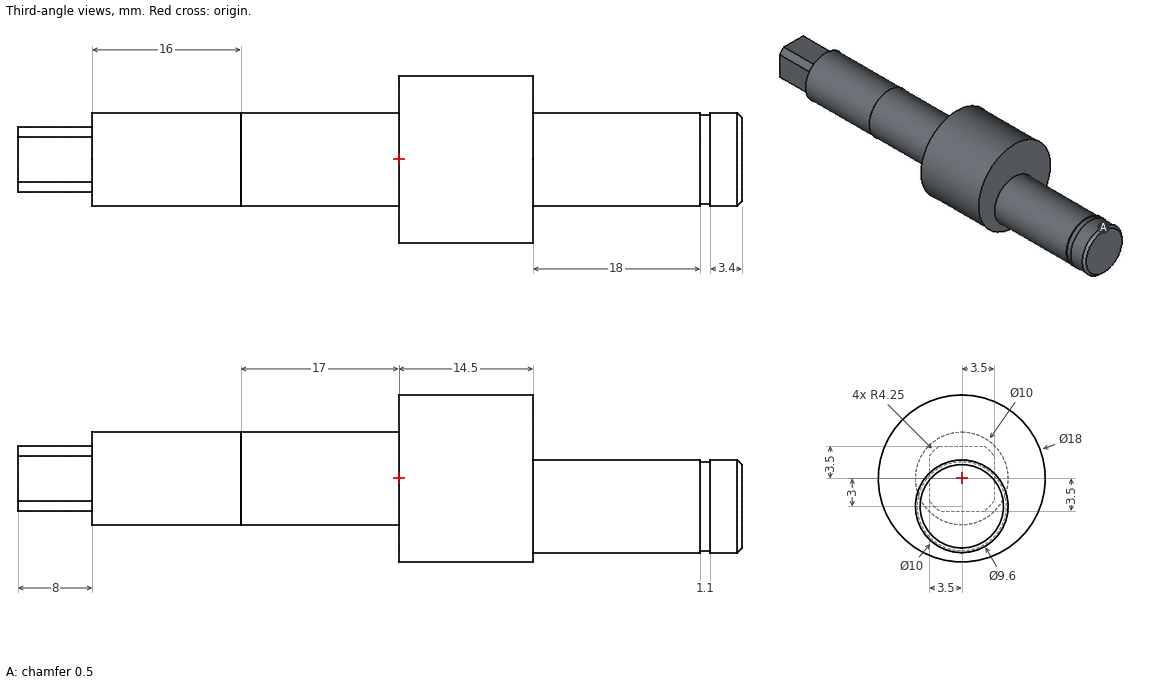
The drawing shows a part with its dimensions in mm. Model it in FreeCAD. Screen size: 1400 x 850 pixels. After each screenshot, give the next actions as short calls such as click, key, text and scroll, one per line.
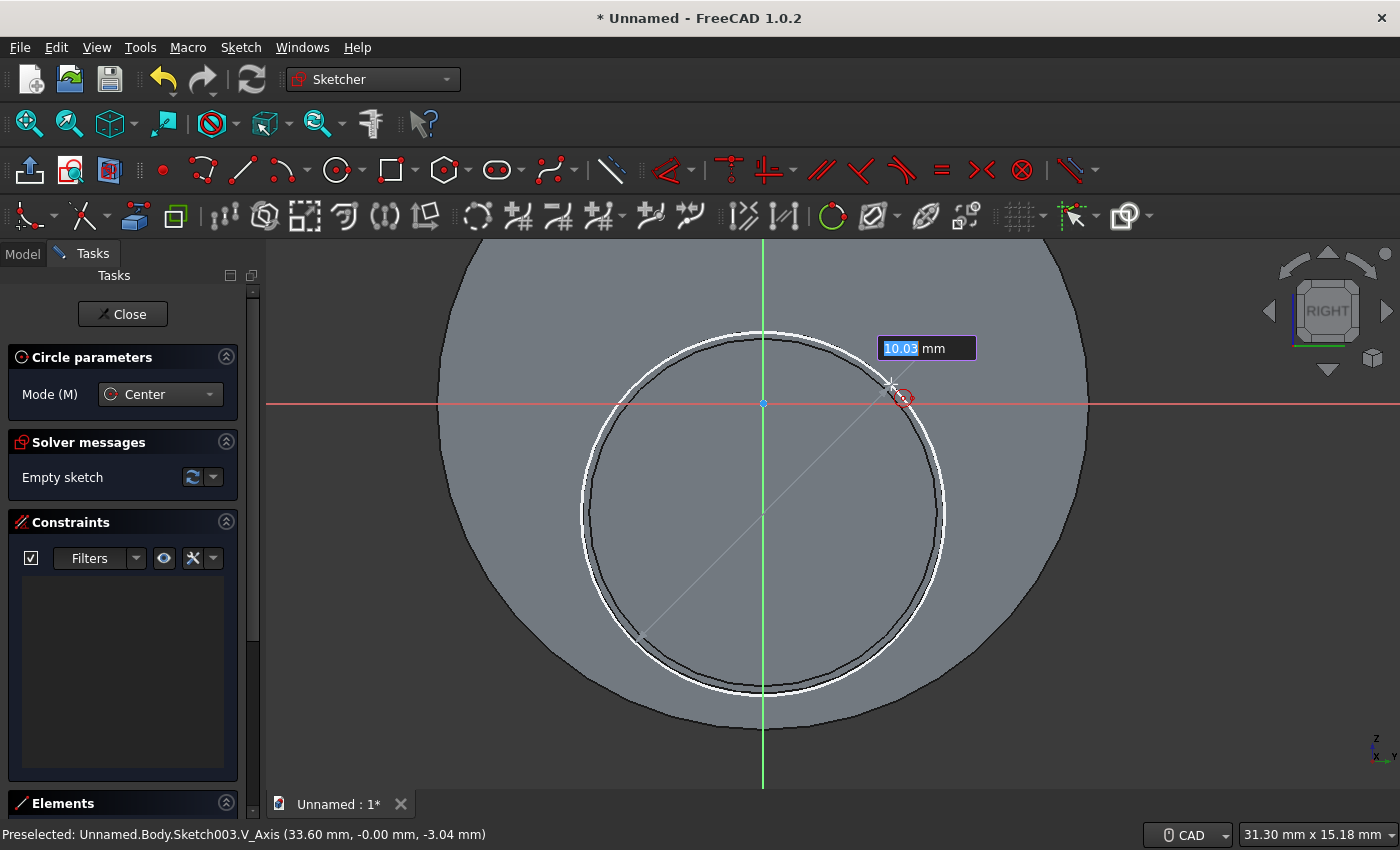
text(10)
key(Return)
key(Escape)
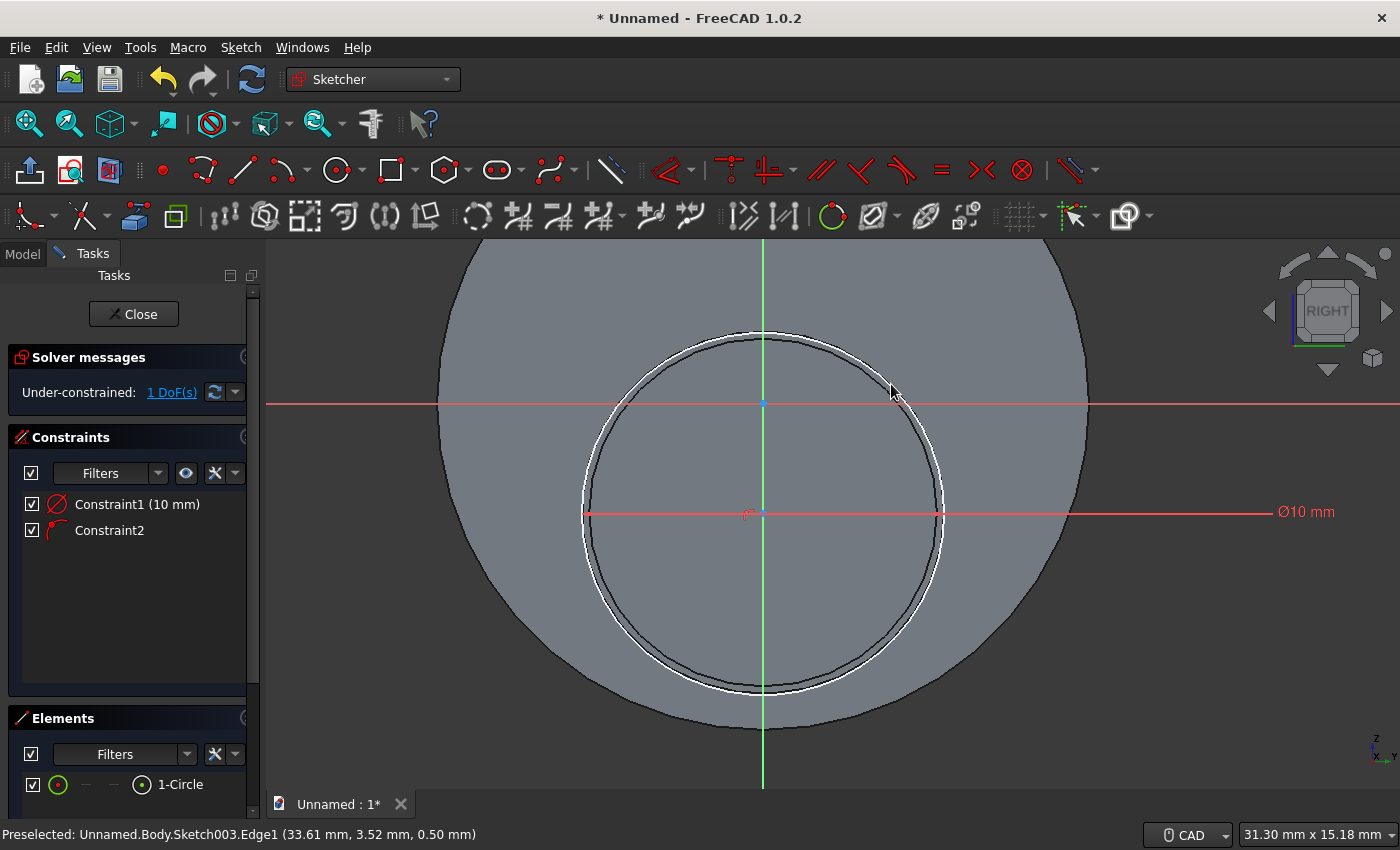
click(666, 170)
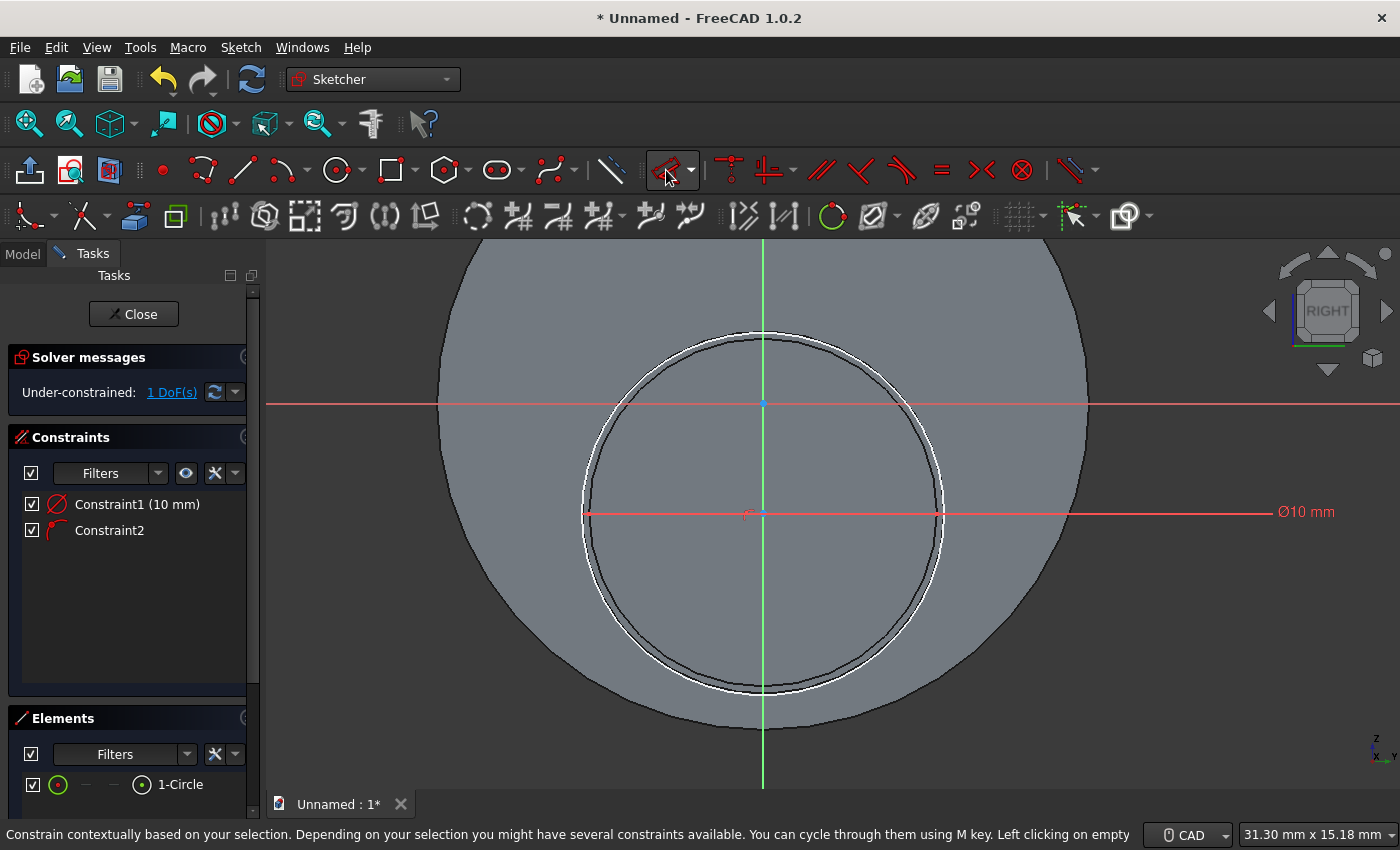
click(763, 514)
click(797, 459)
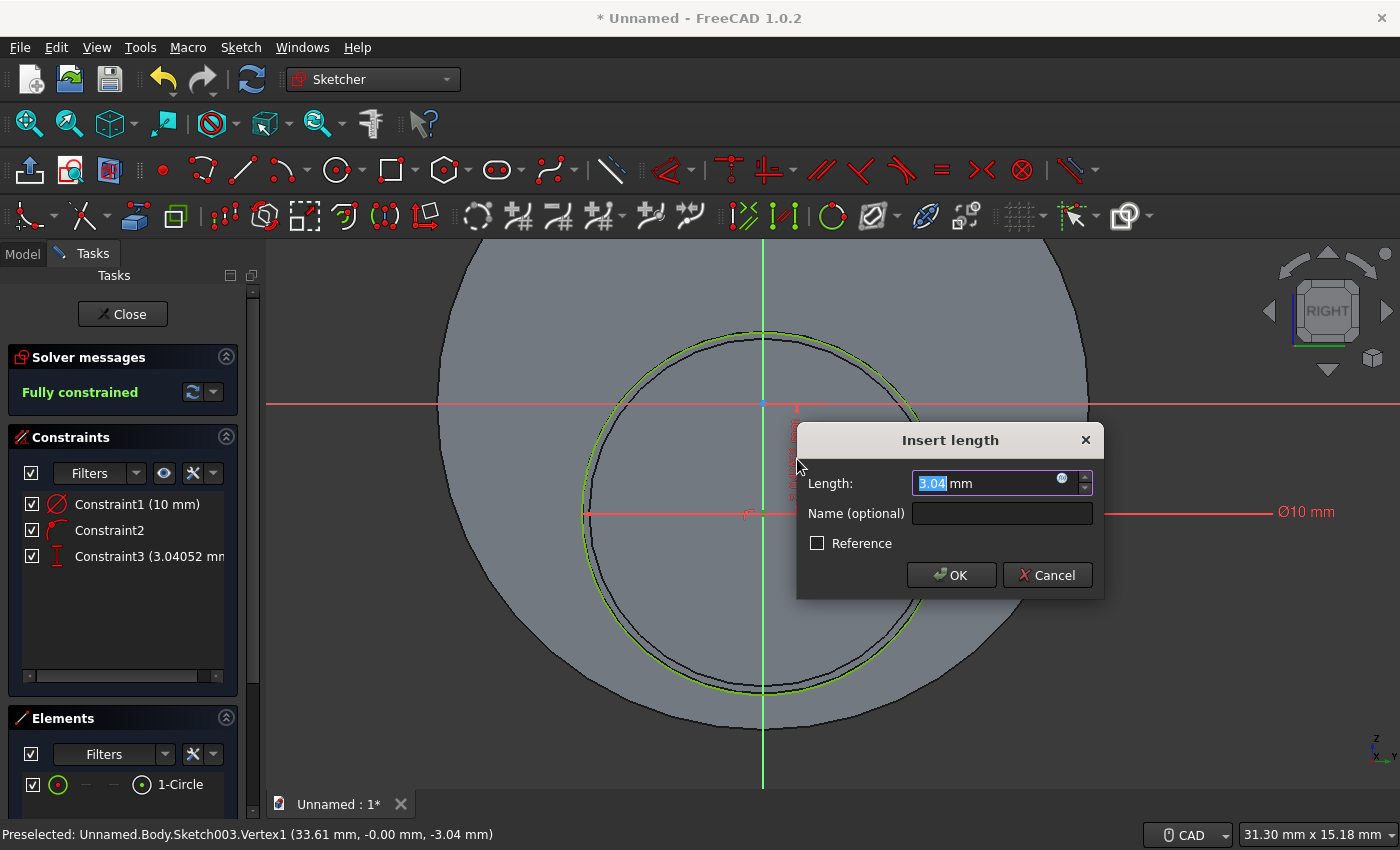
text(3)
key(Return)
key(Escape)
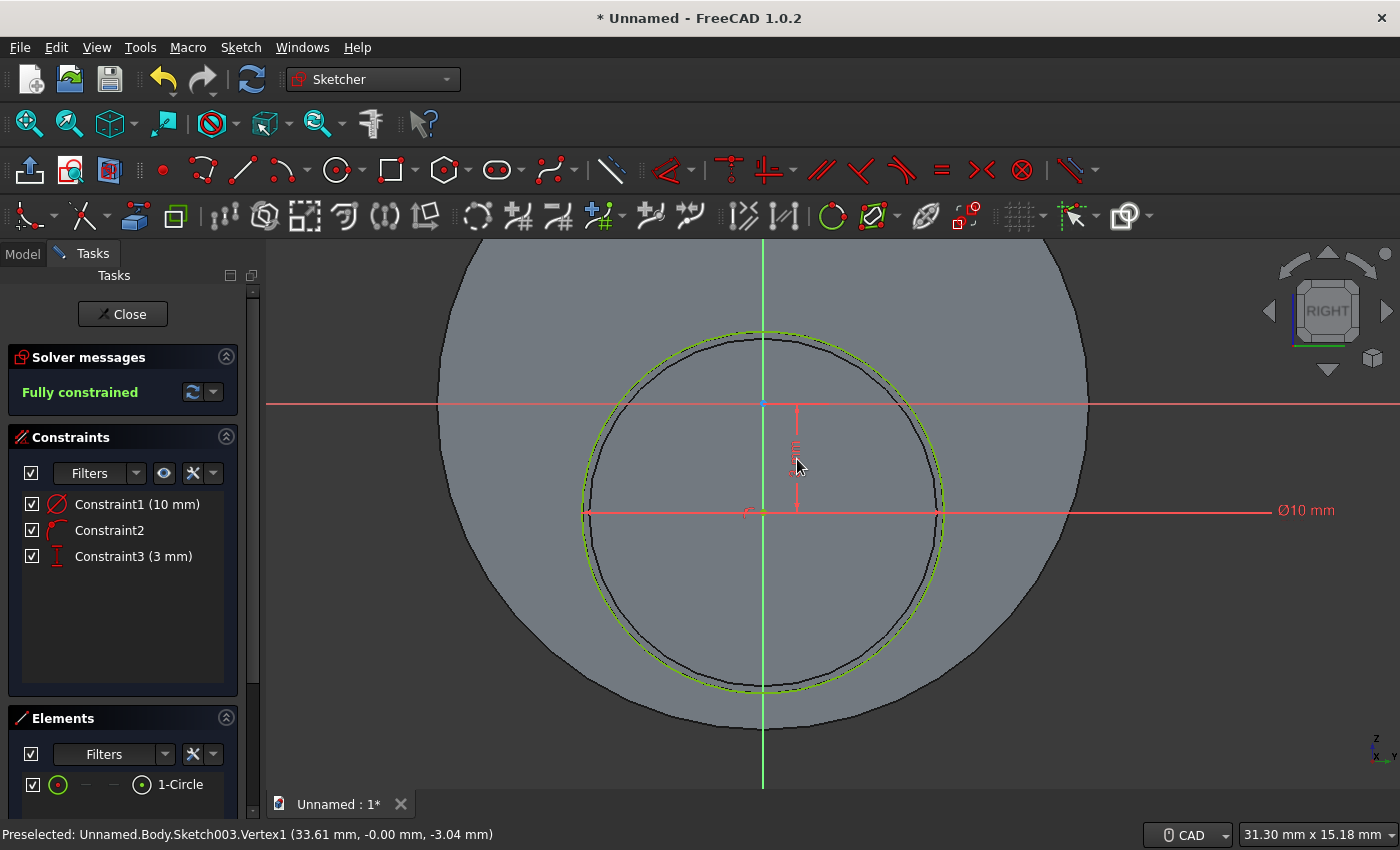
click(123, 314)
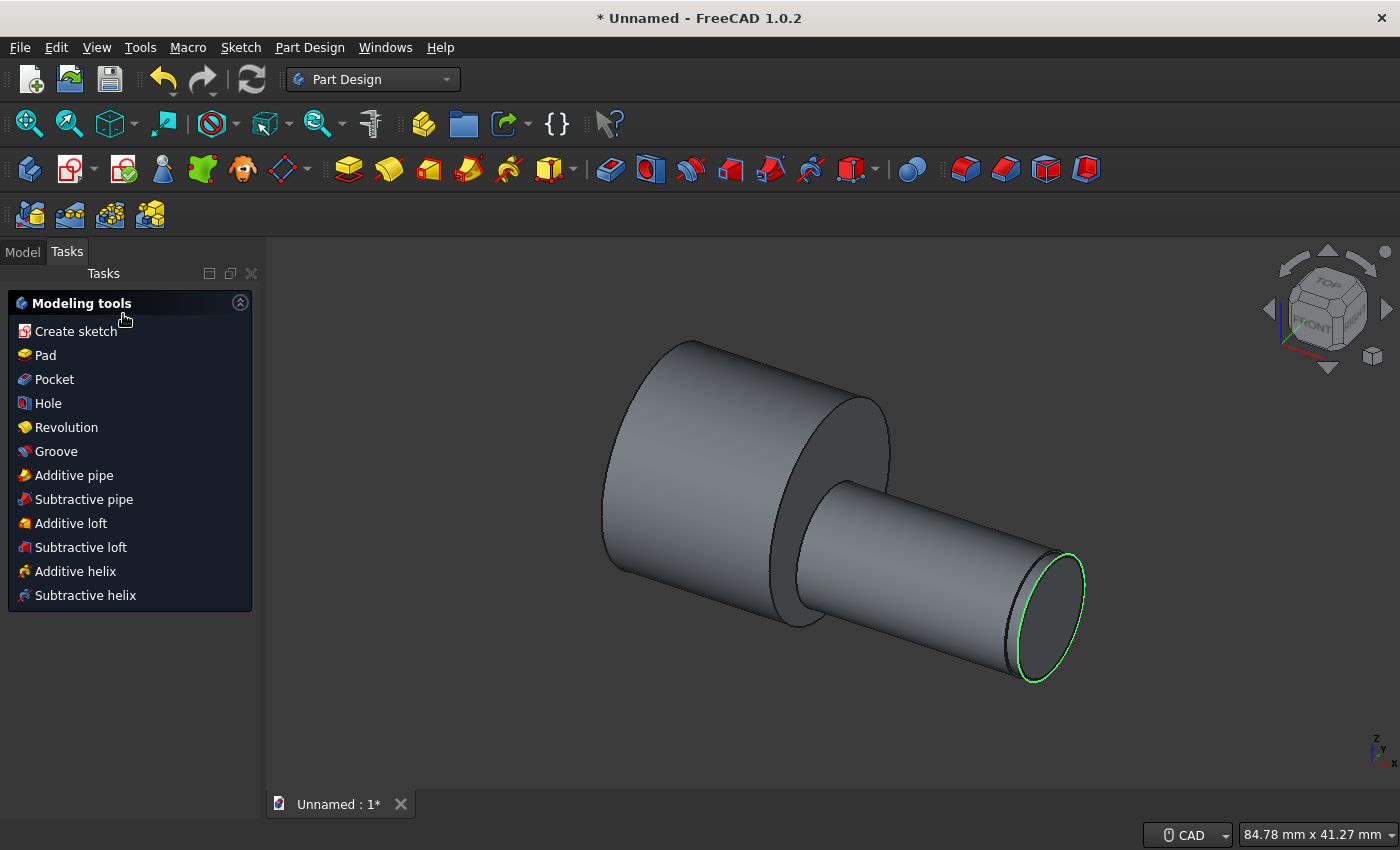
click(350, 170)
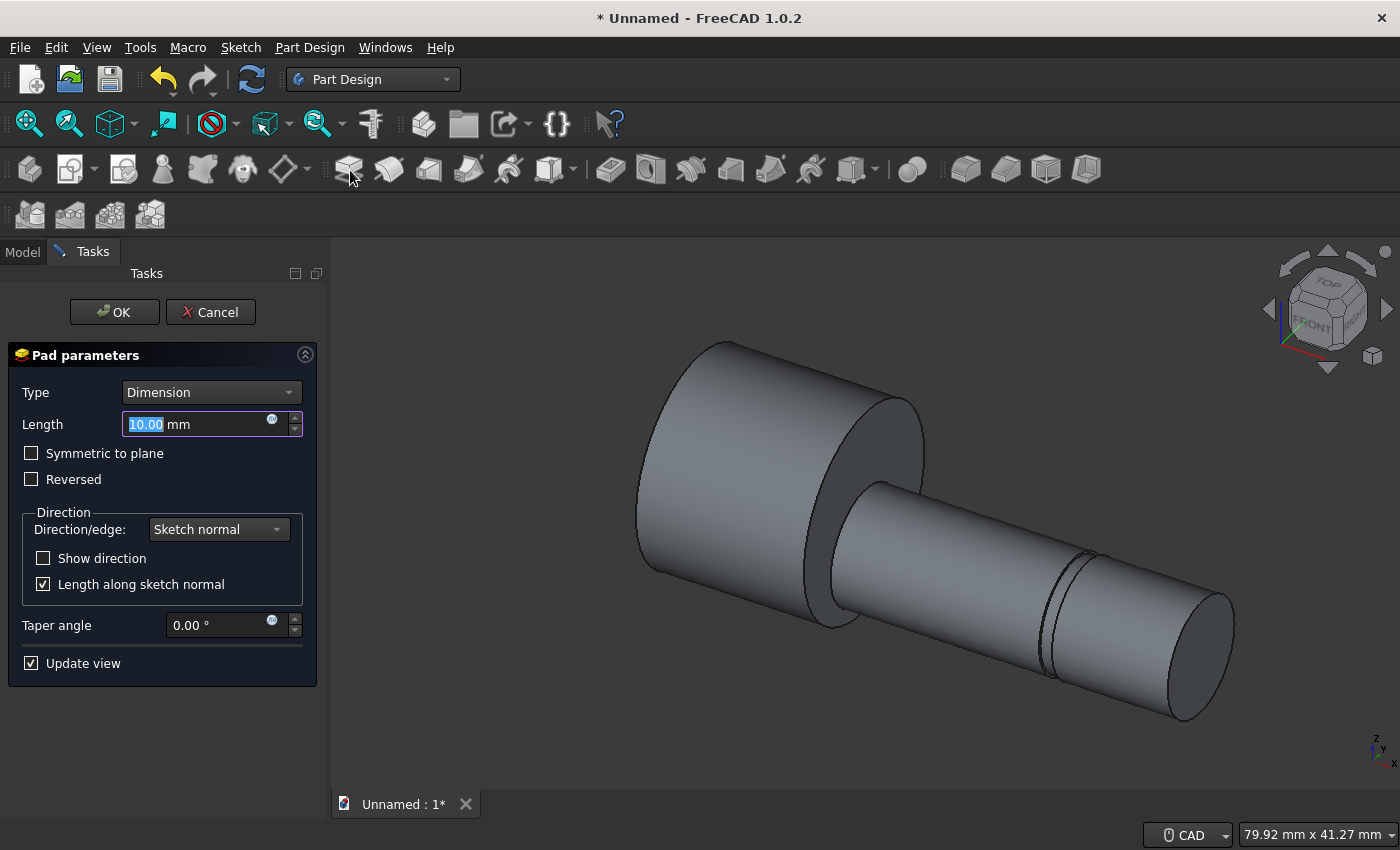
text(3.4)
key(Tab)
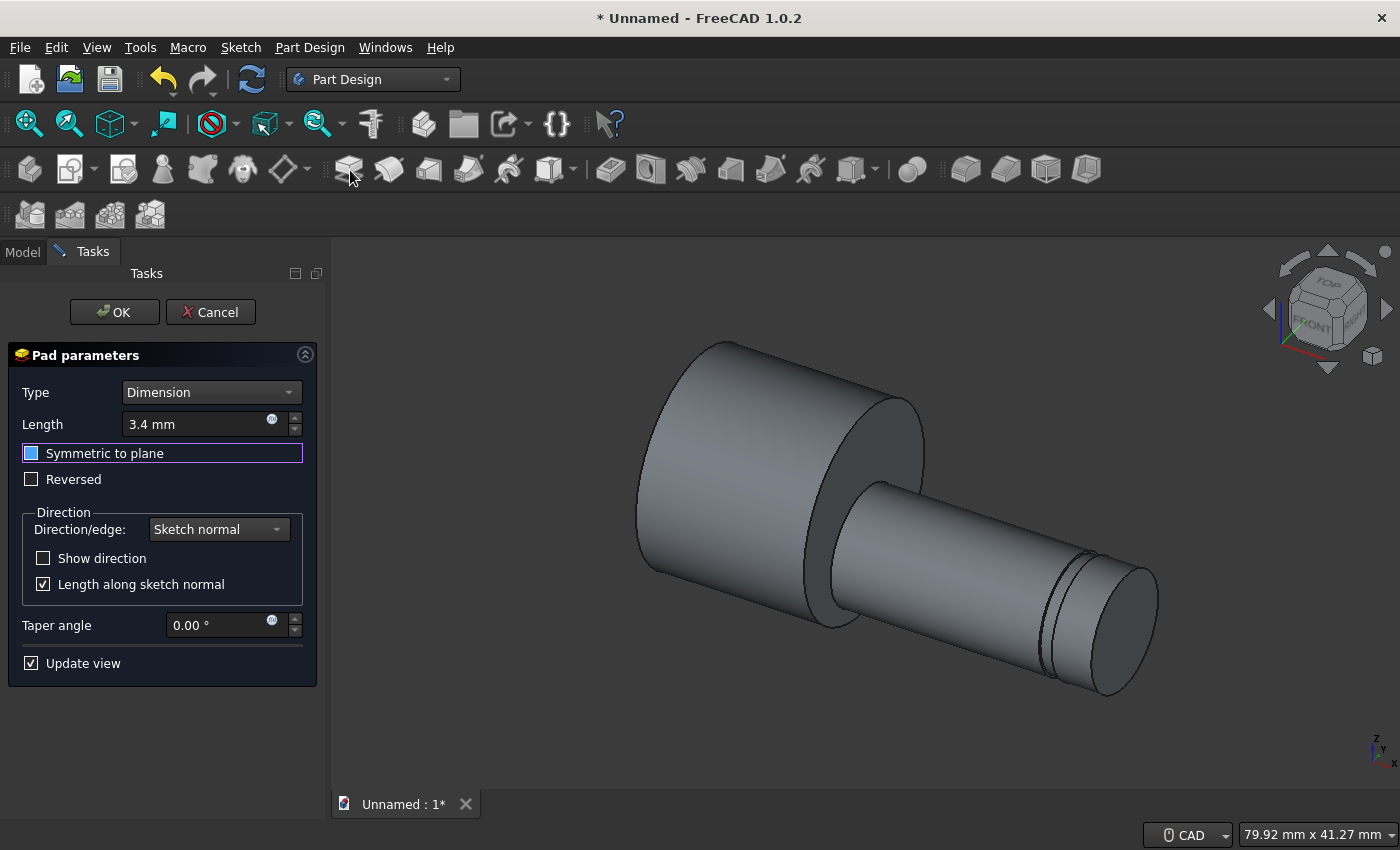
click(115, 312)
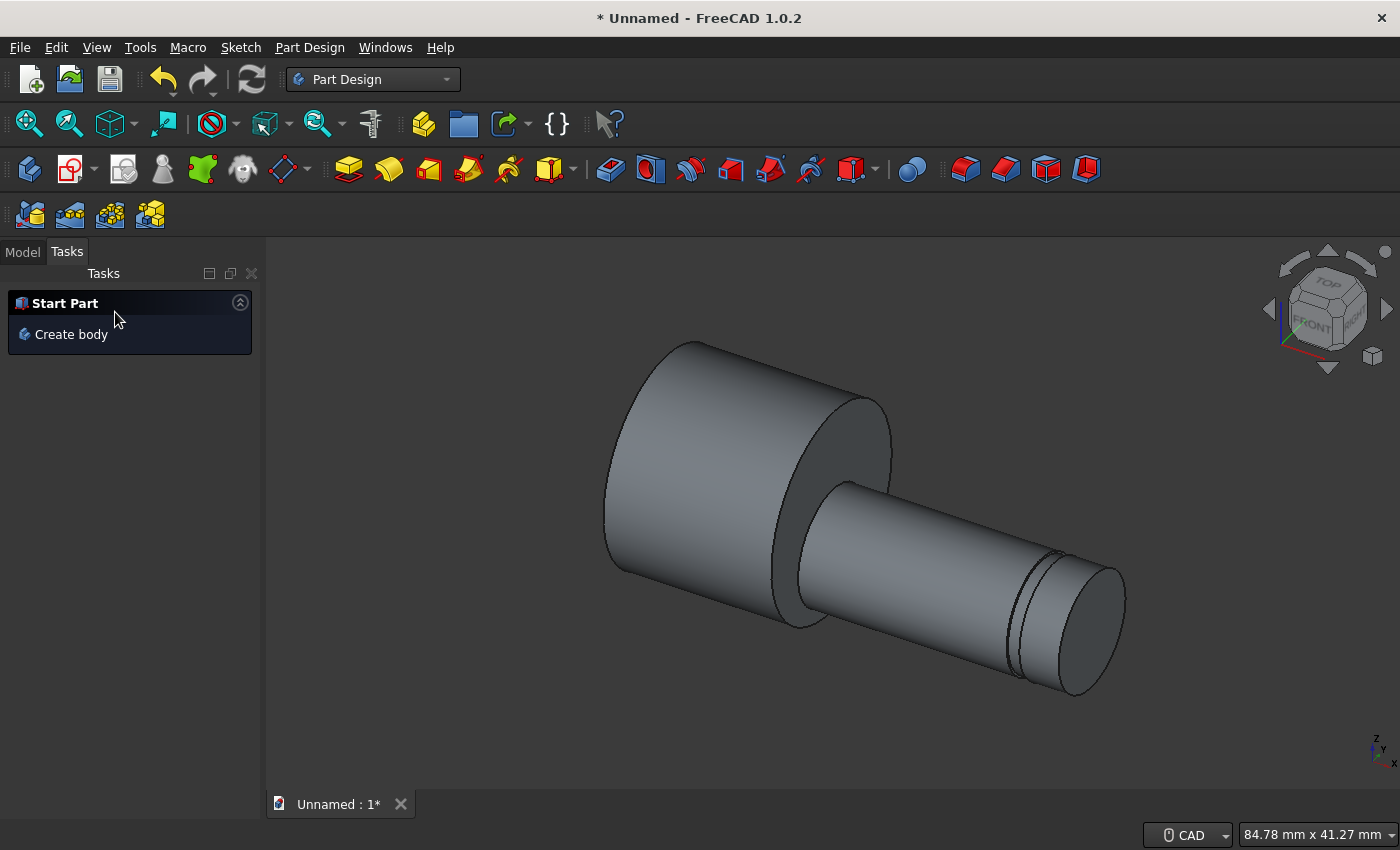
click(1059, 664)